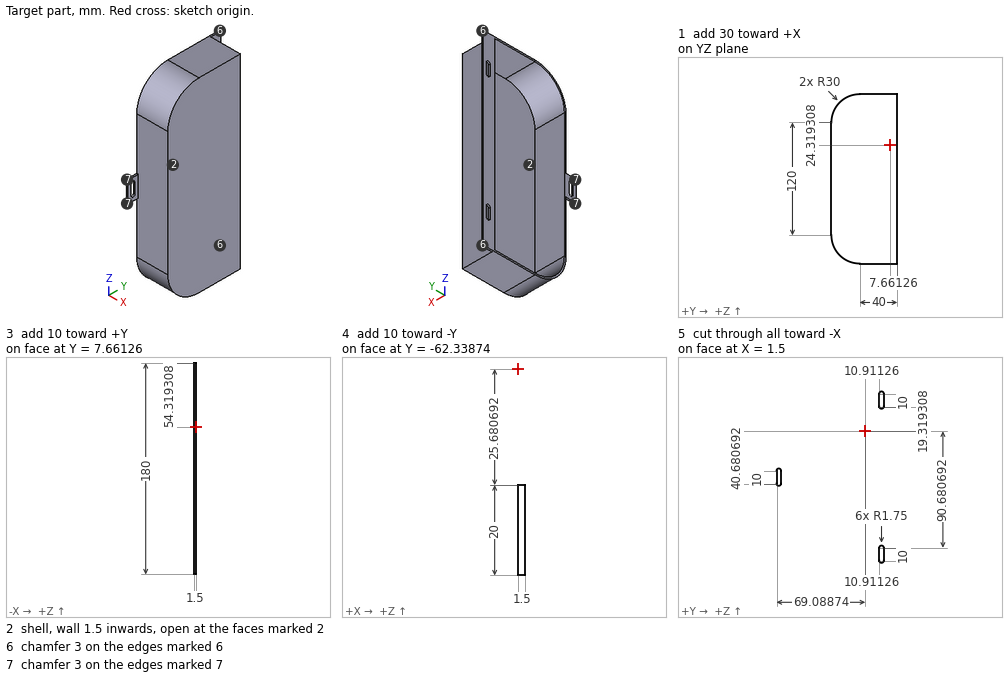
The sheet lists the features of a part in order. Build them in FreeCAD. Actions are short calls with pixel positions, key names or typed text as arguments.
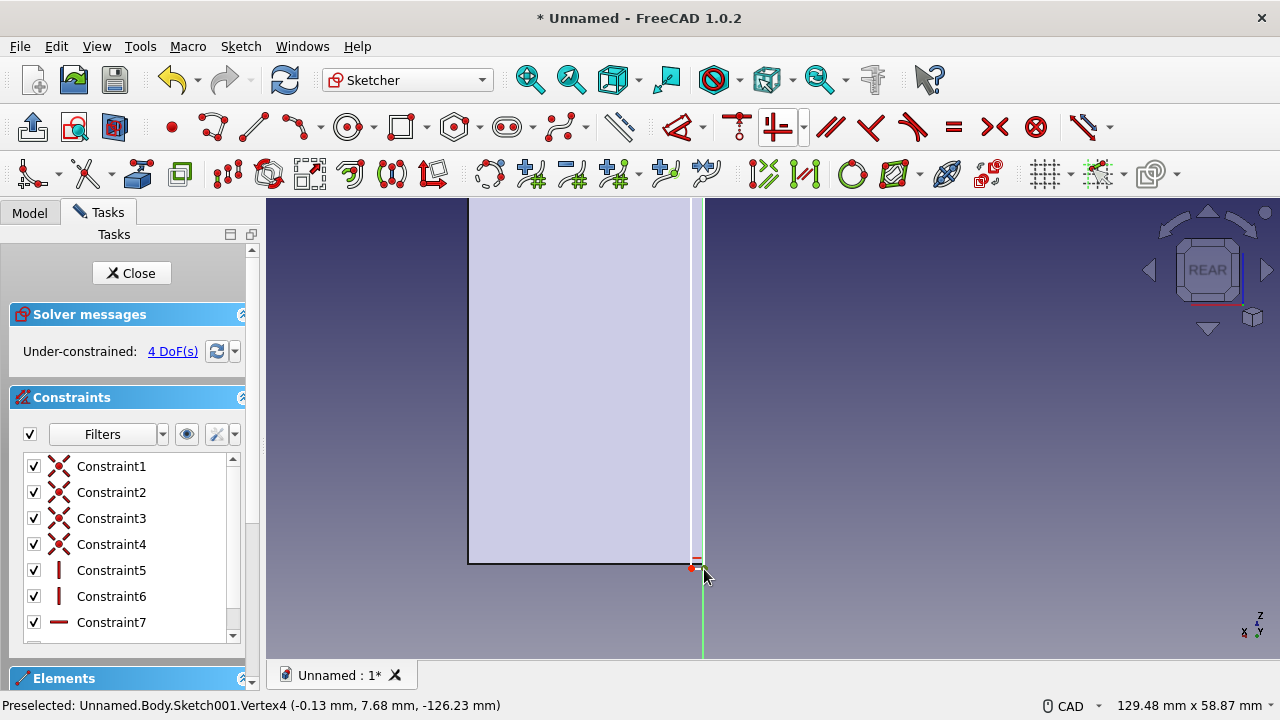
click(703, 602)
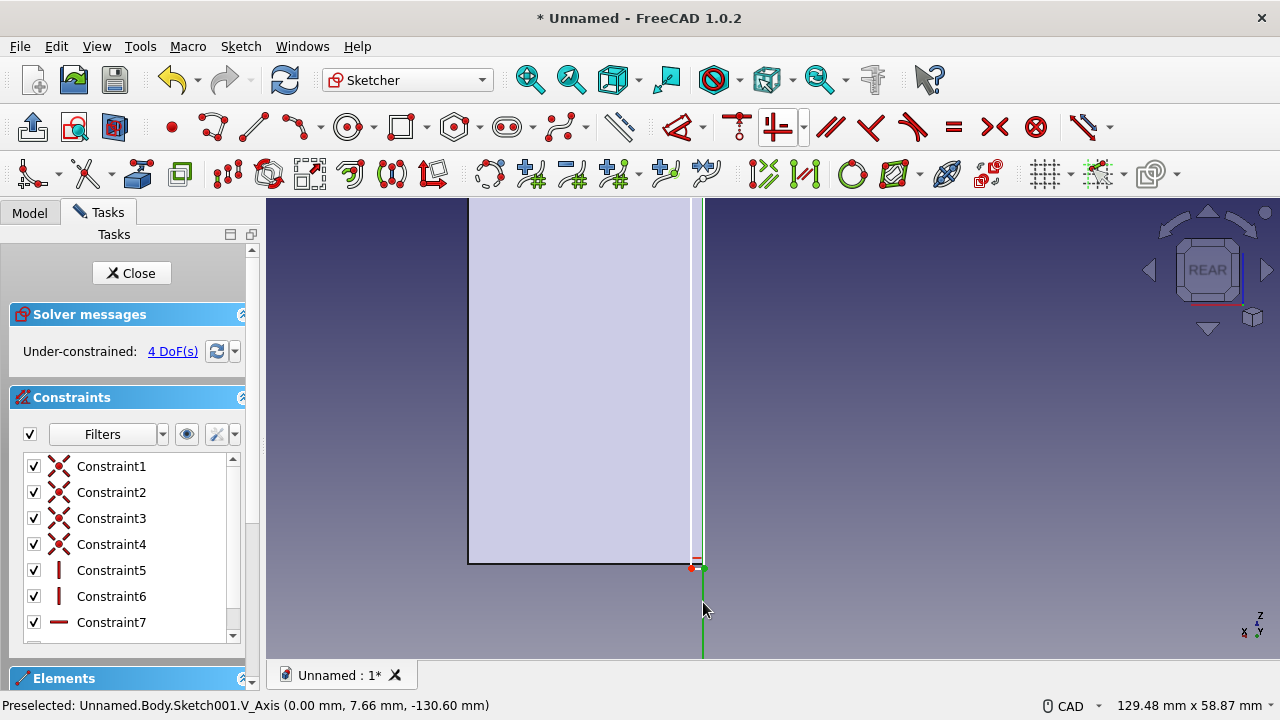
click(737, 128)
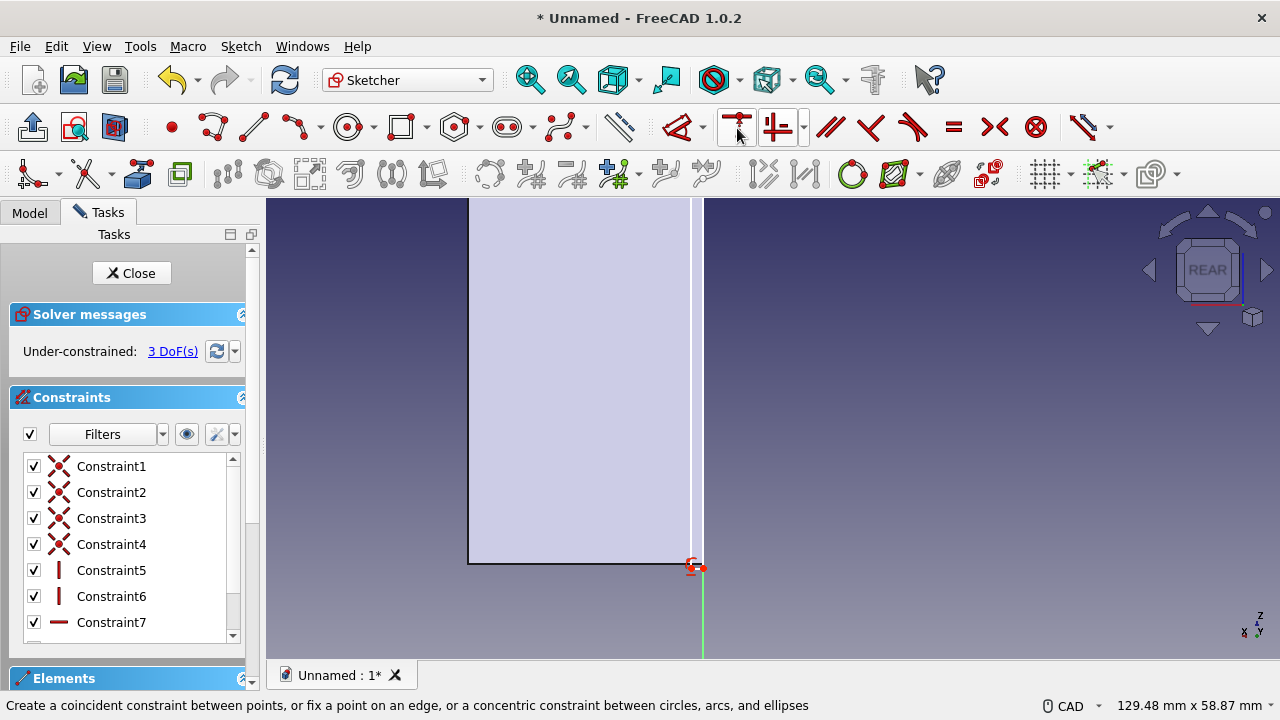
click(676, 128)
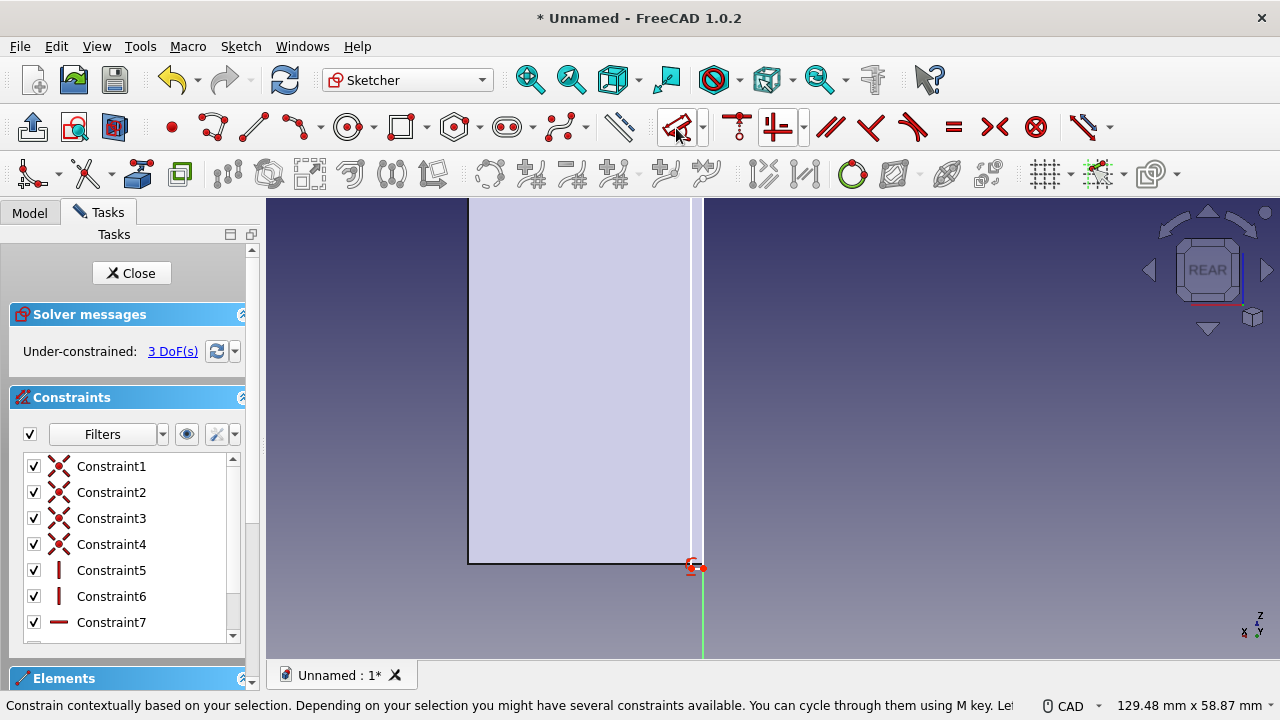
click(691, 286)
click(657, 397)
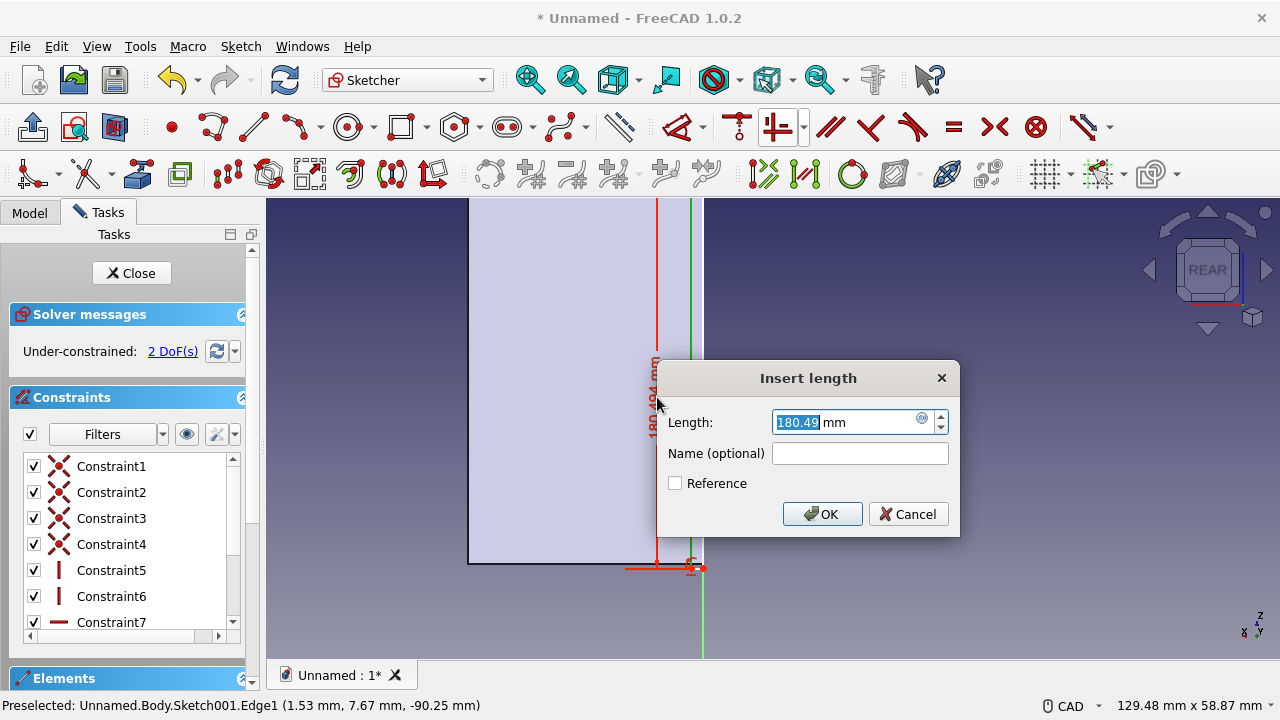
text(180)
key(Return)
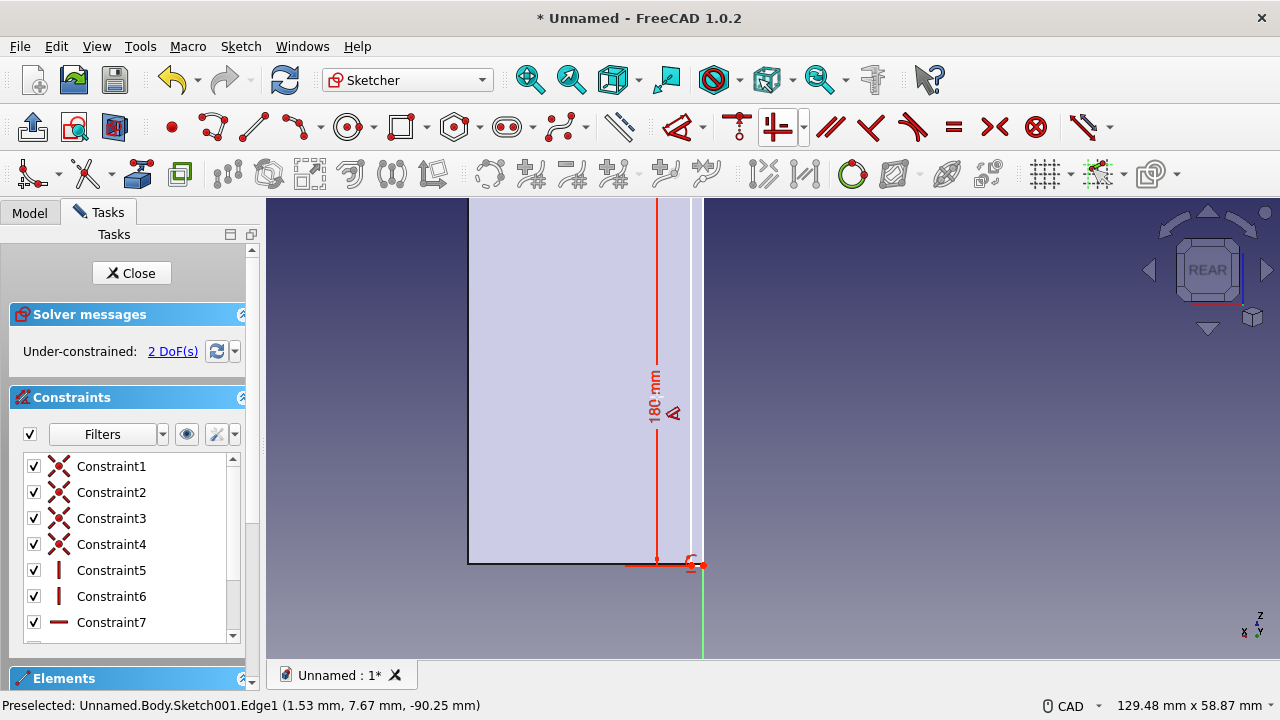
scroll(697, 566, up, 7)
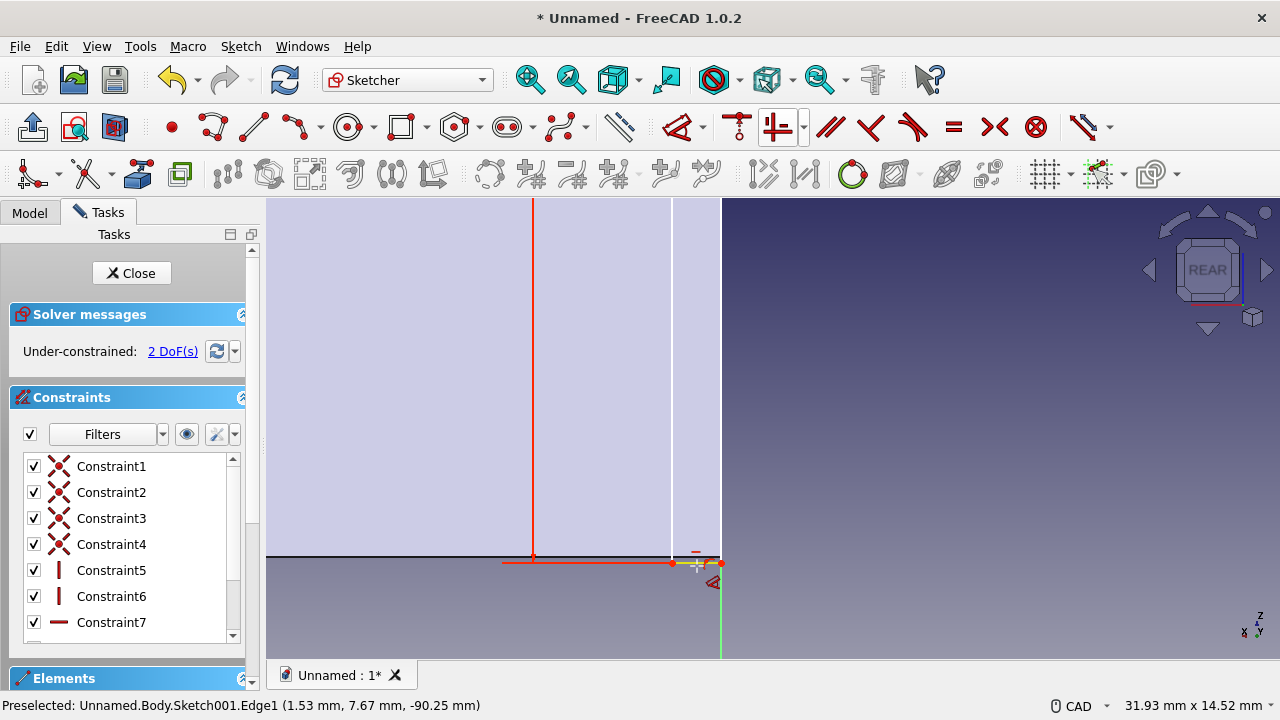
click(697, 563)
click(697, 597)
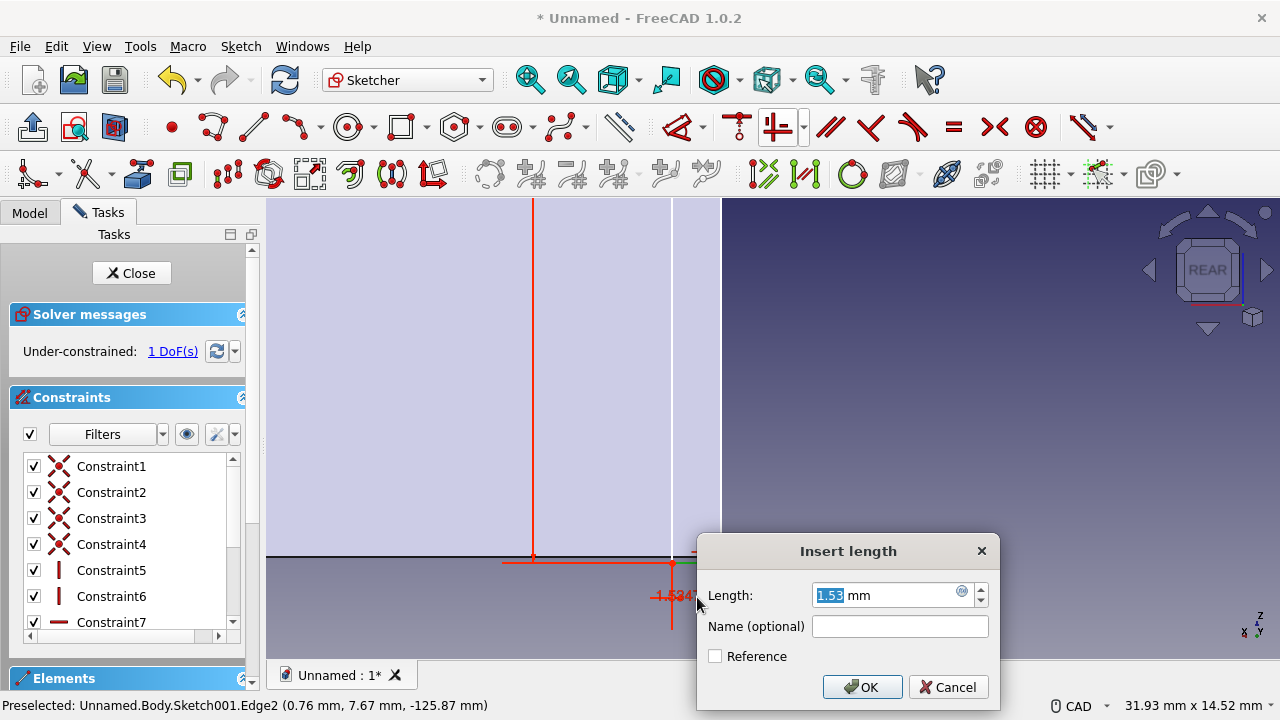
text(1.5)
key(Return)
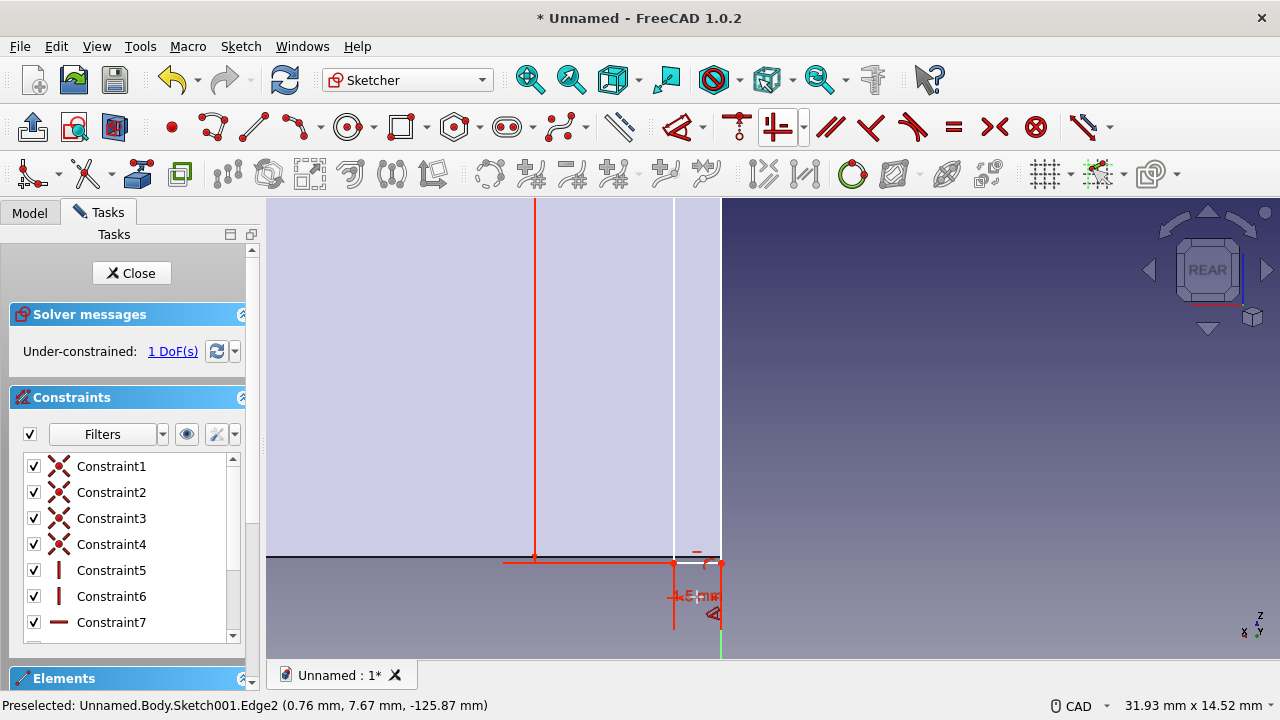
scroll(705, 572, down, 15)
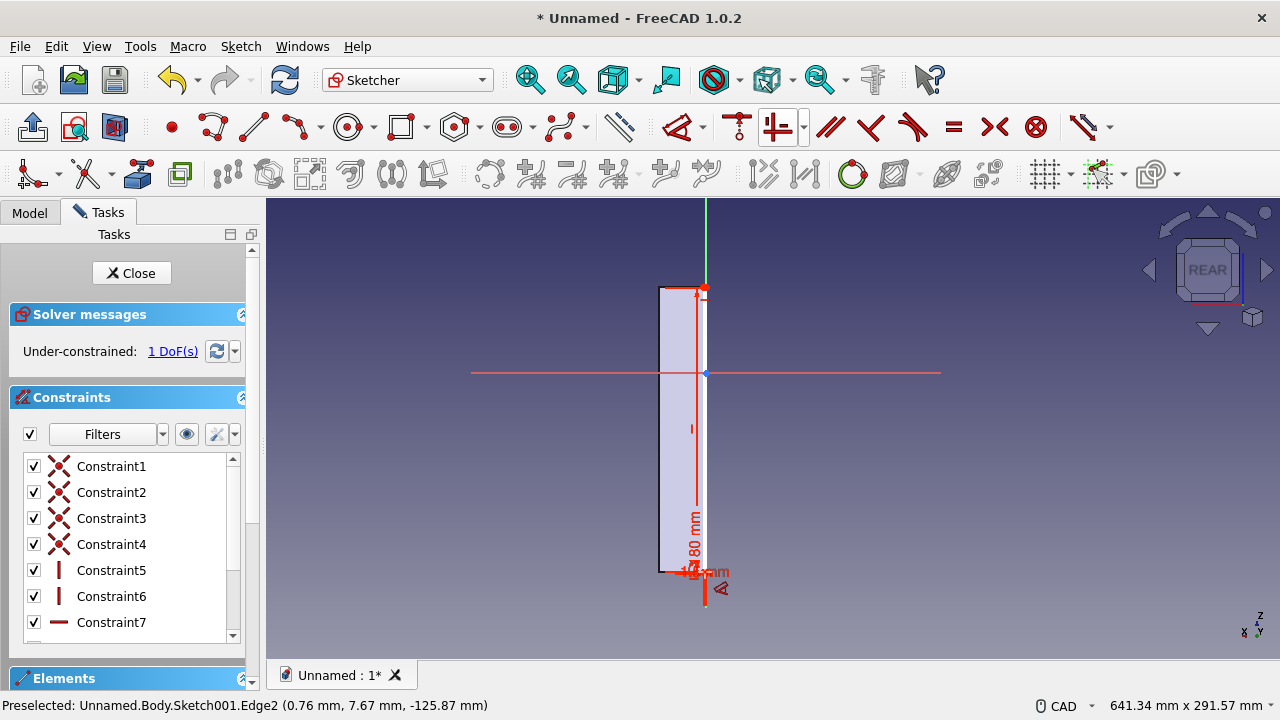
scroll(704, 288, up, 9)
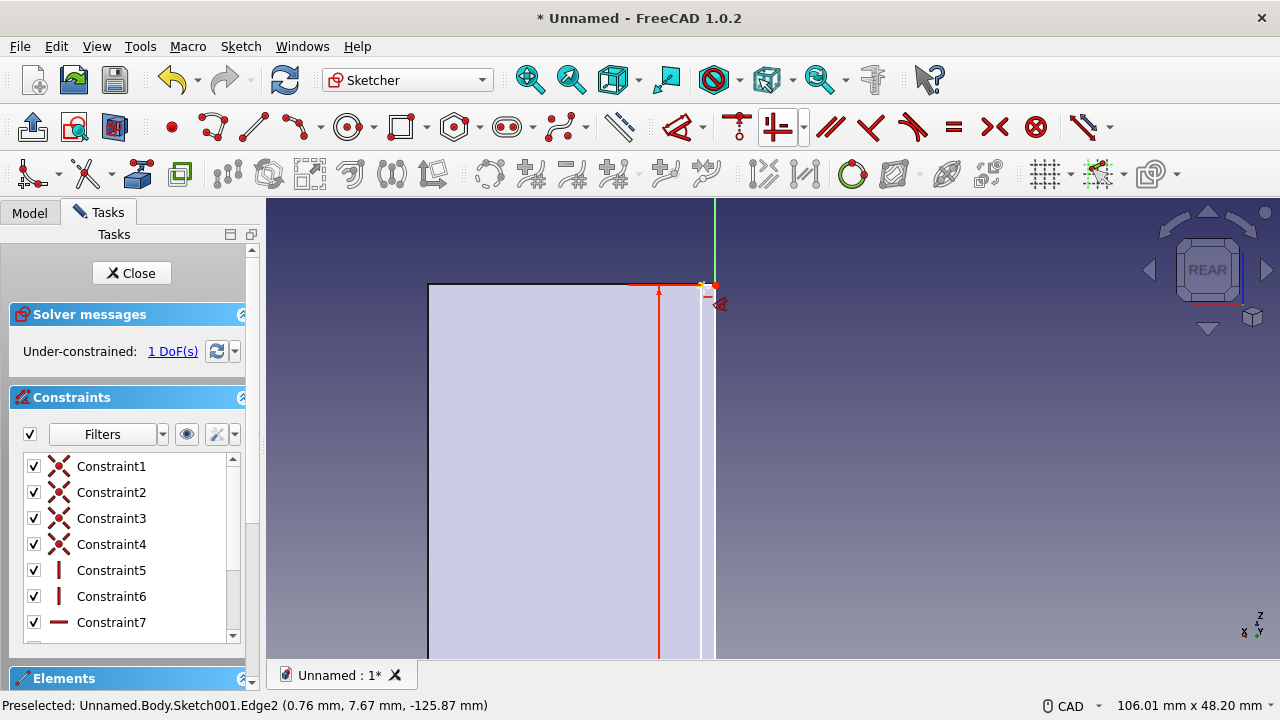
click(701, 285)
click(749, 458)